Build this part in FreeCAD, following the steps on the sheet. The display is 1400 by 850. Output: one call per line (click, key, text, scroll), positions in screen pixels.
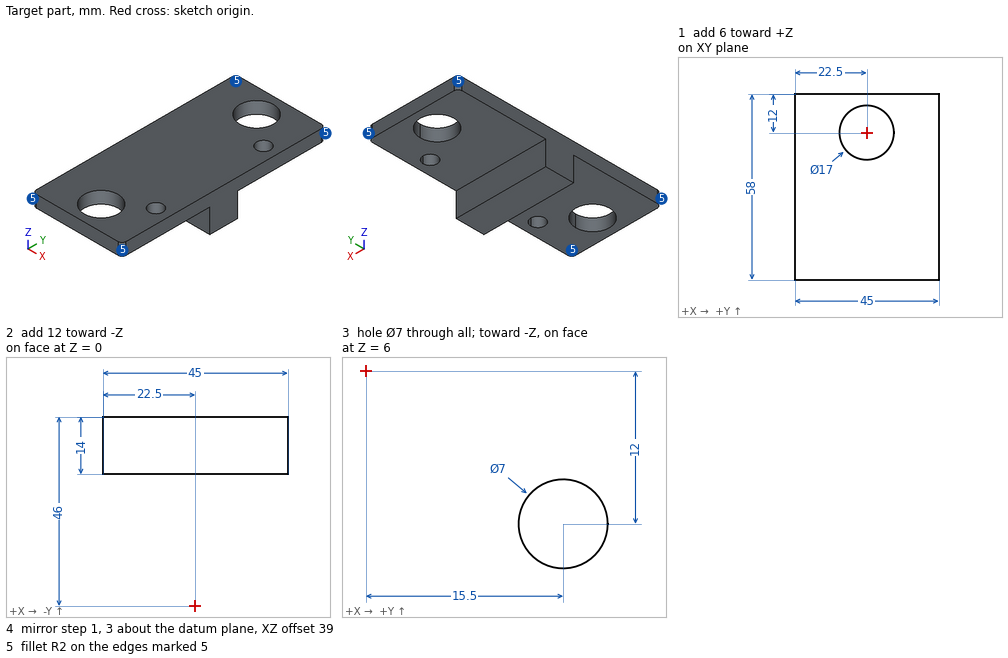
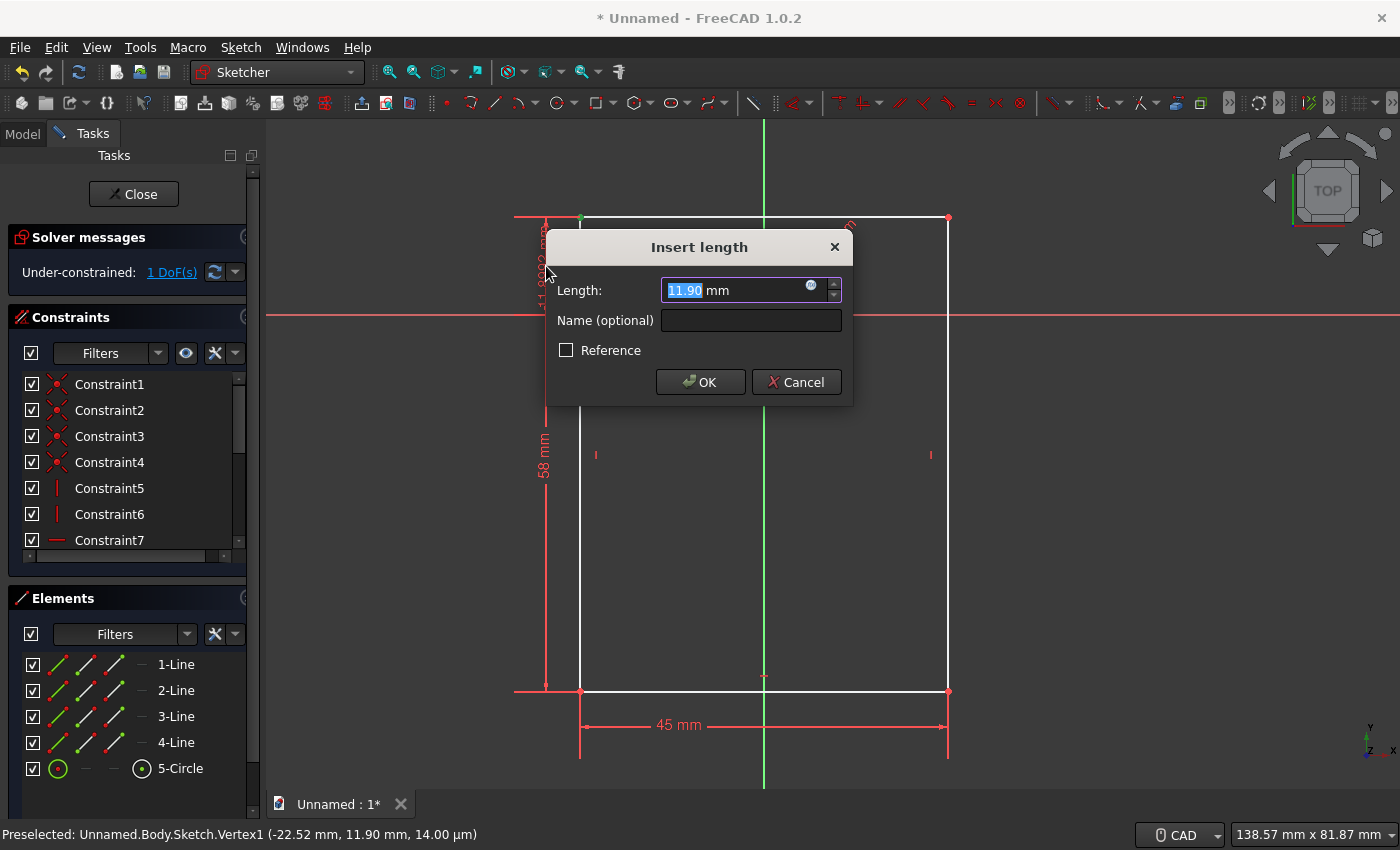
text(12)
key(Return)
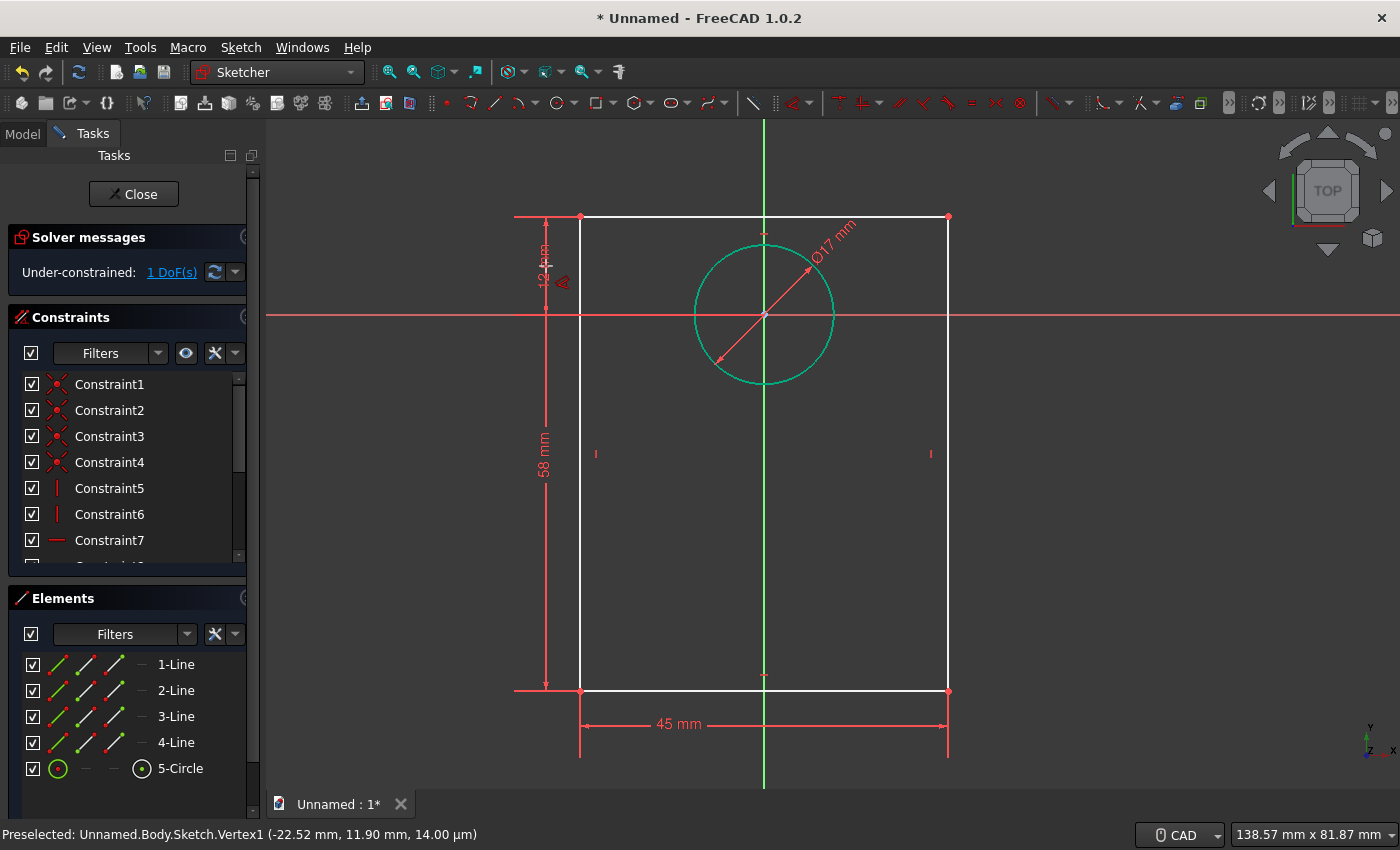
click(580, 217)
click(672, 183)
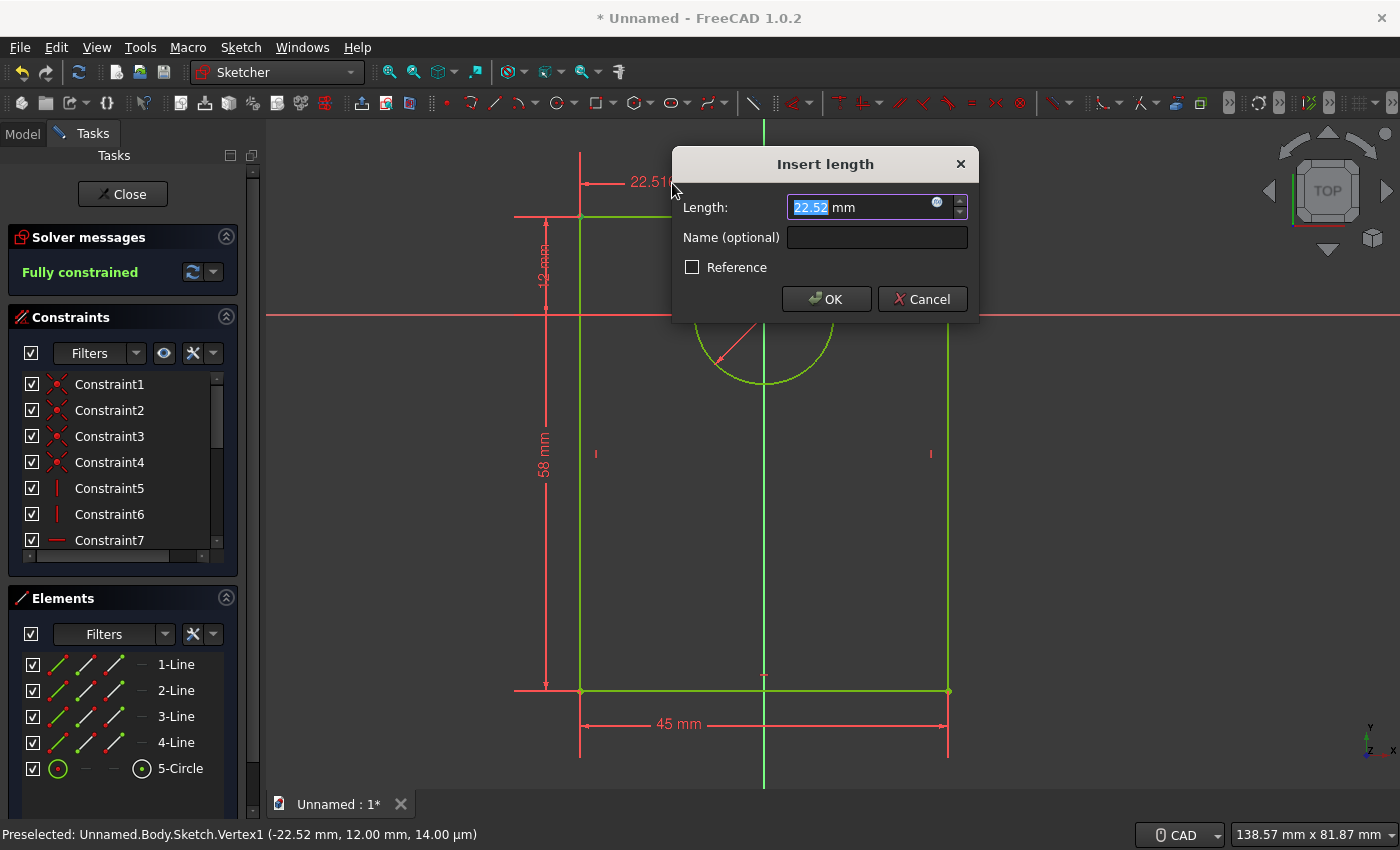
text(22.5)
key(Return)
key(Escape)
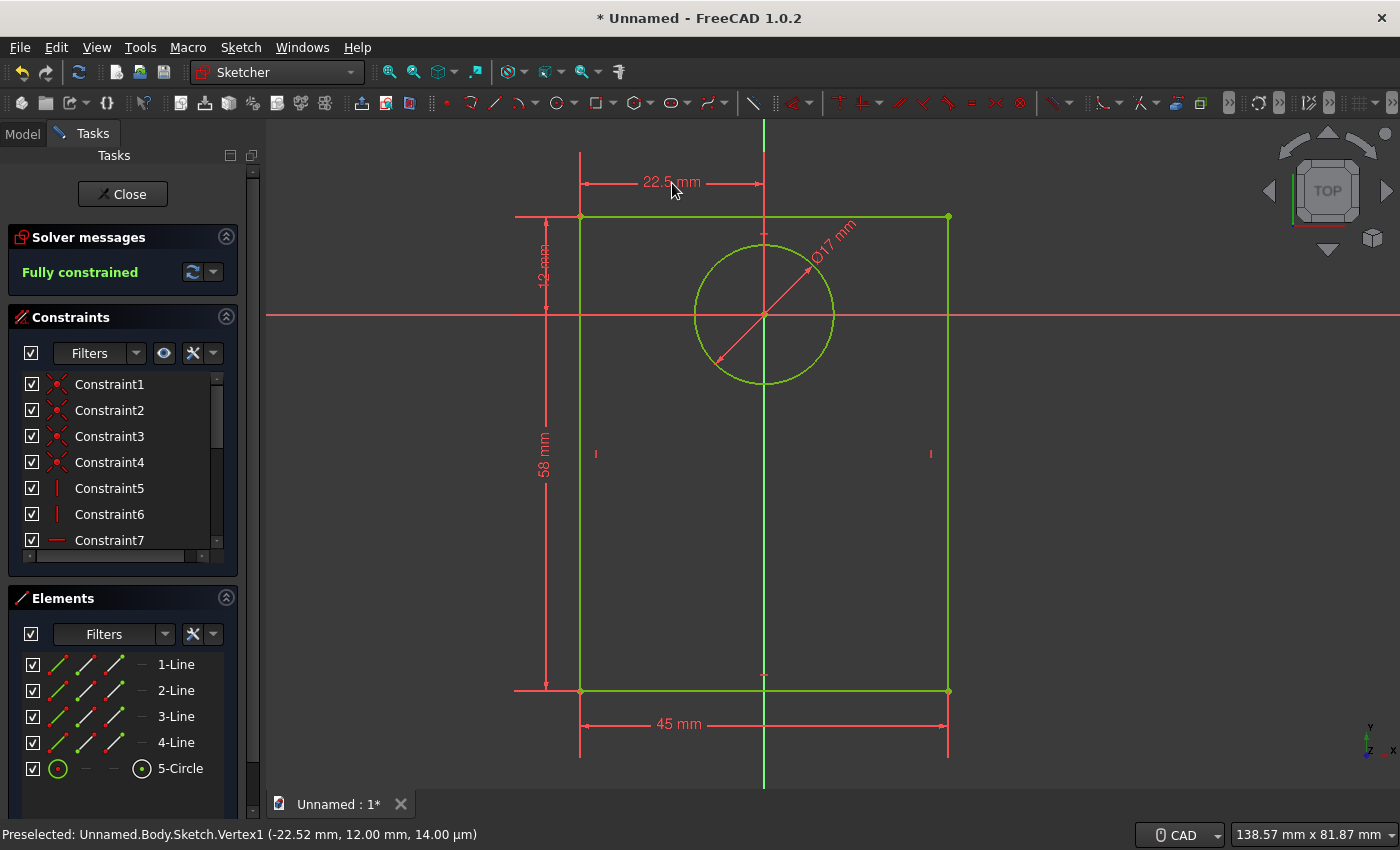
click(123, 194)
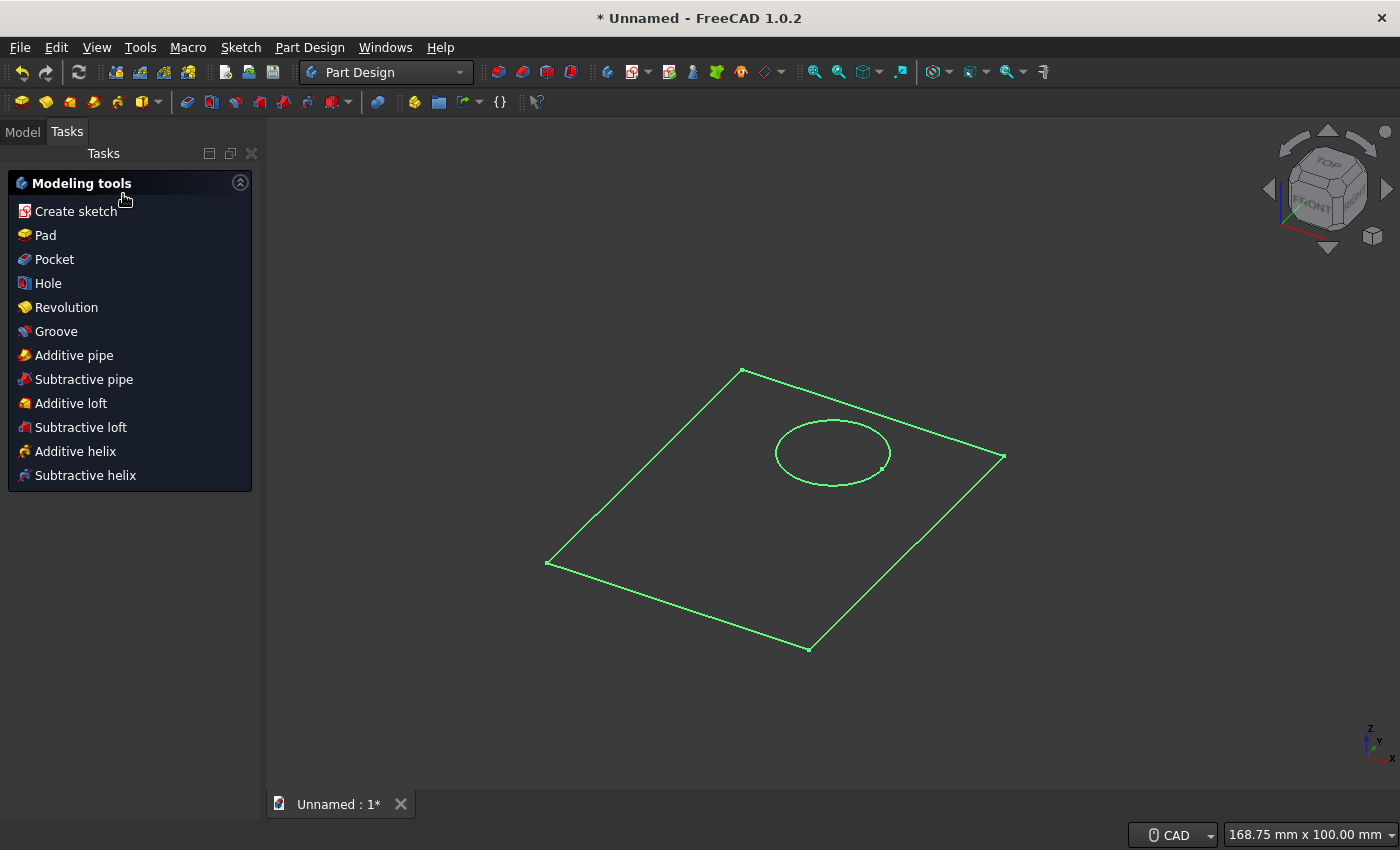
click(22, 102)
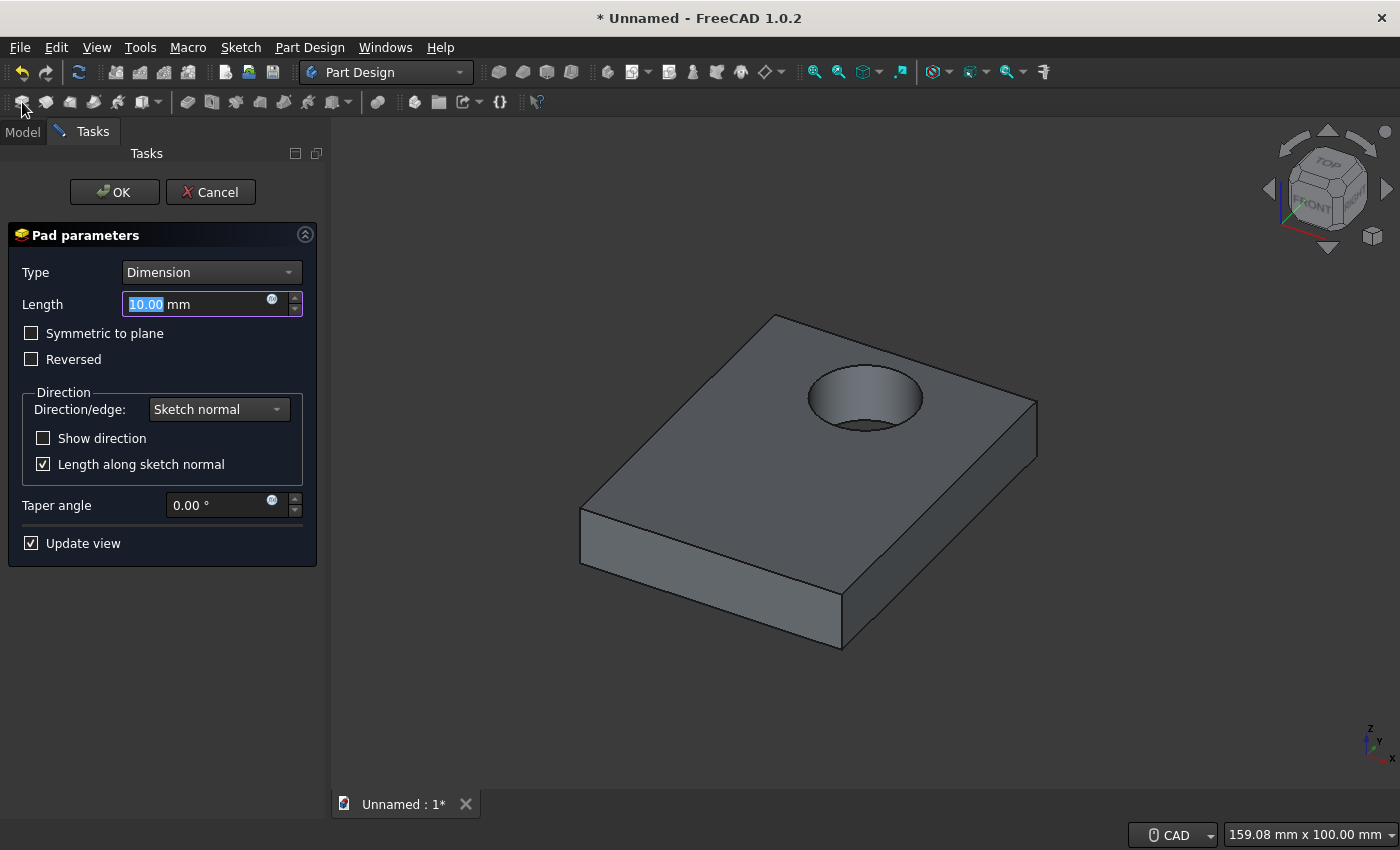
text(6)
key(Tab)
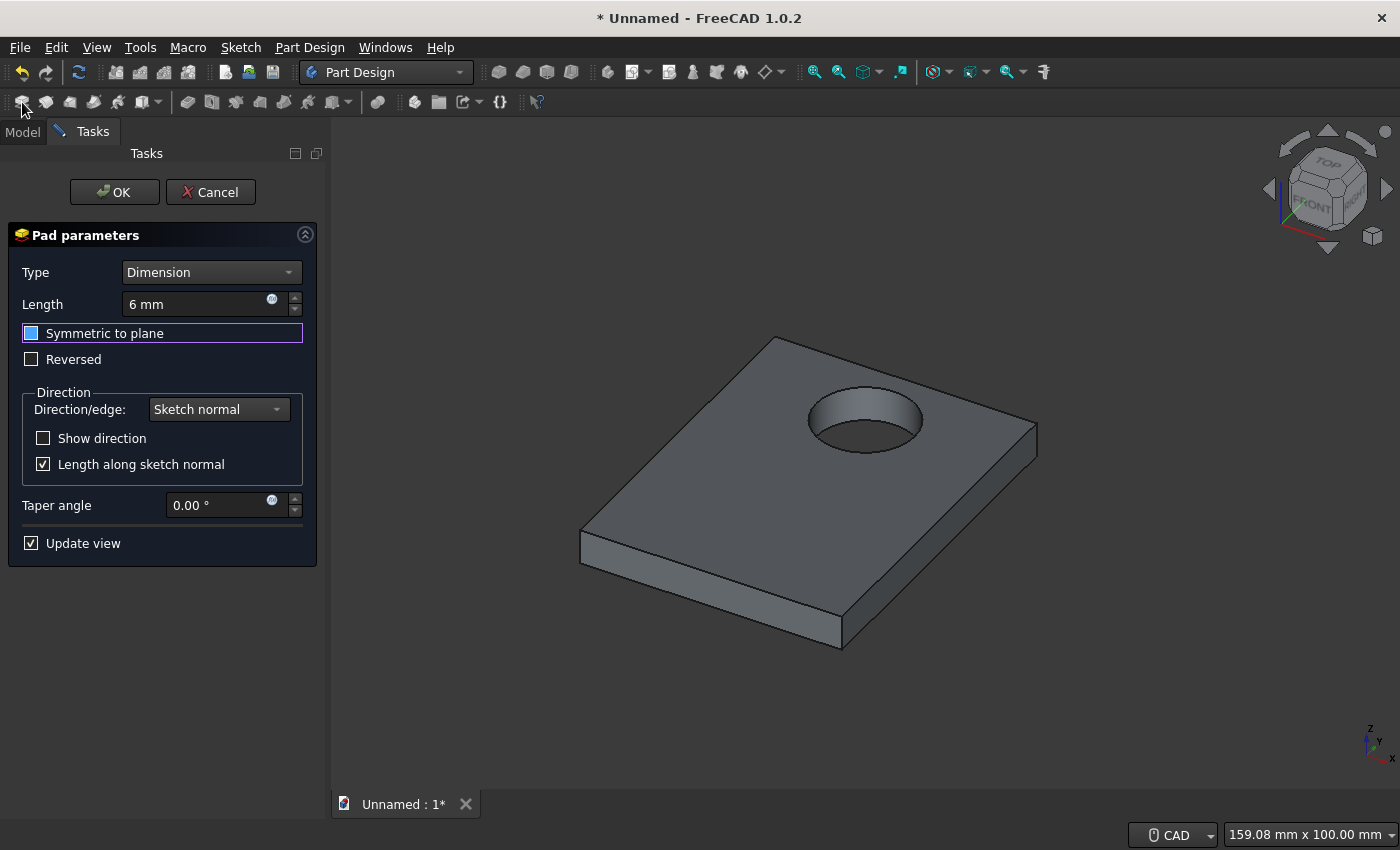
click(115, 192)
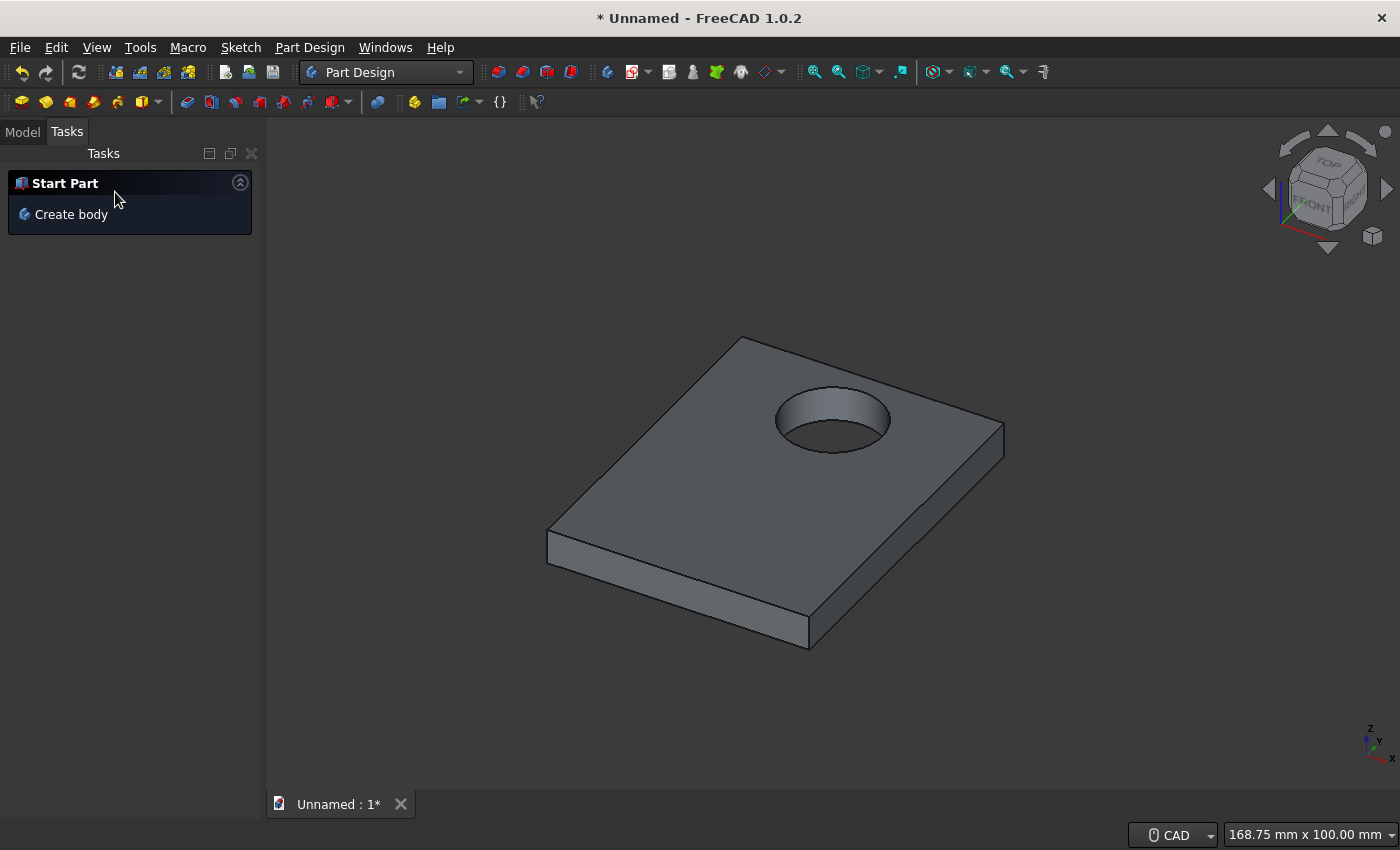
key(5)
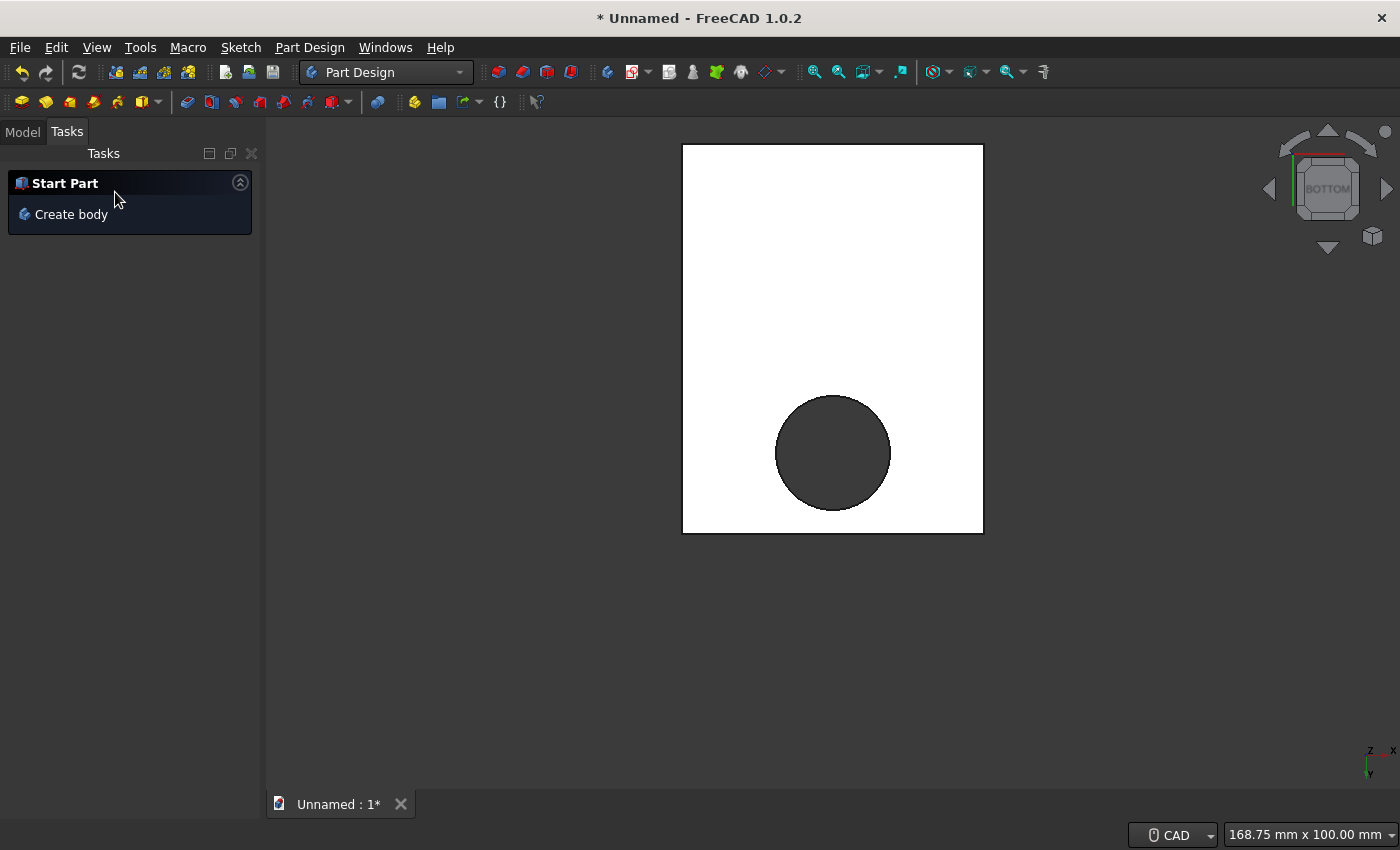
click(833, 282)